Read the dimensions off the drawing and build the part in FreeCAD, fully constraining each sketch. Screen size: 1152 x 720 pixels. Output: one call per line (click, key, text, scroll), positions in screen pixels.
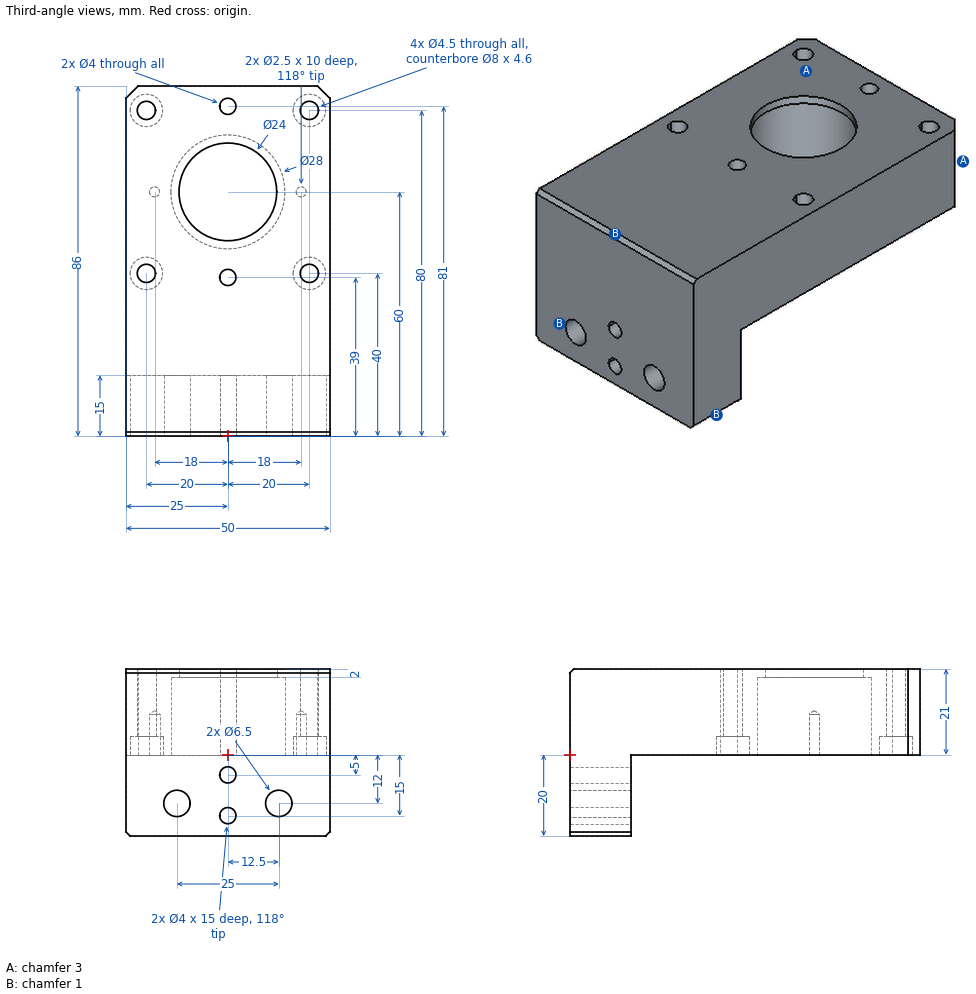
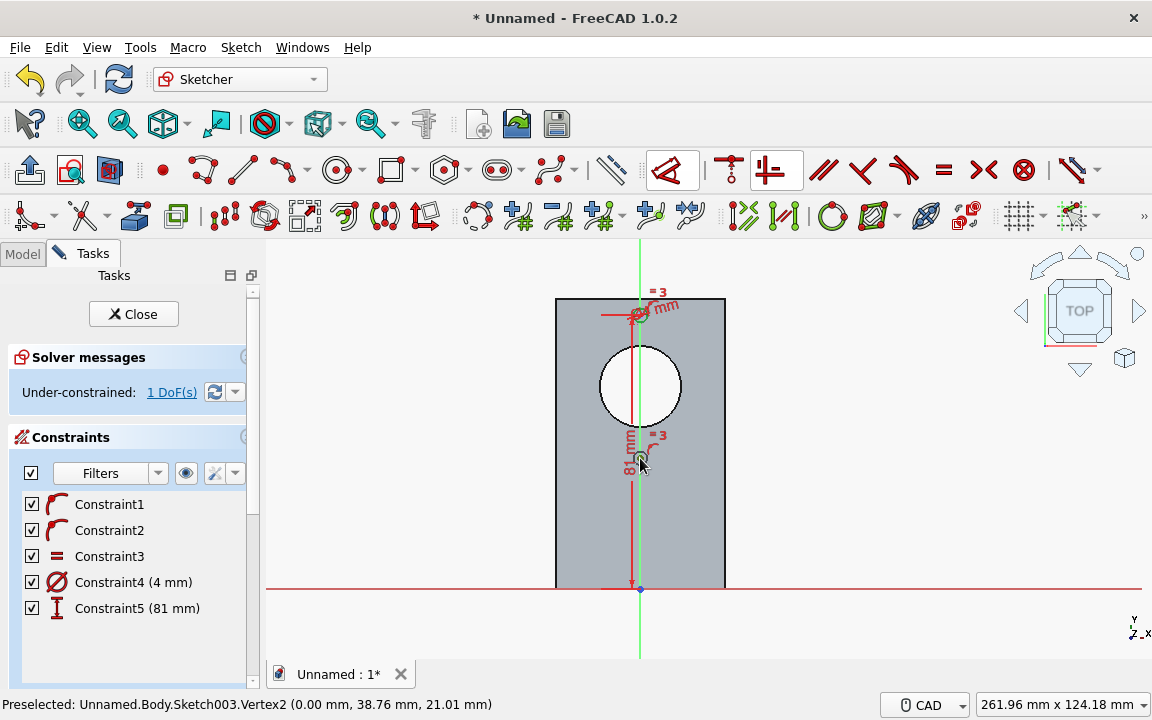
key(i)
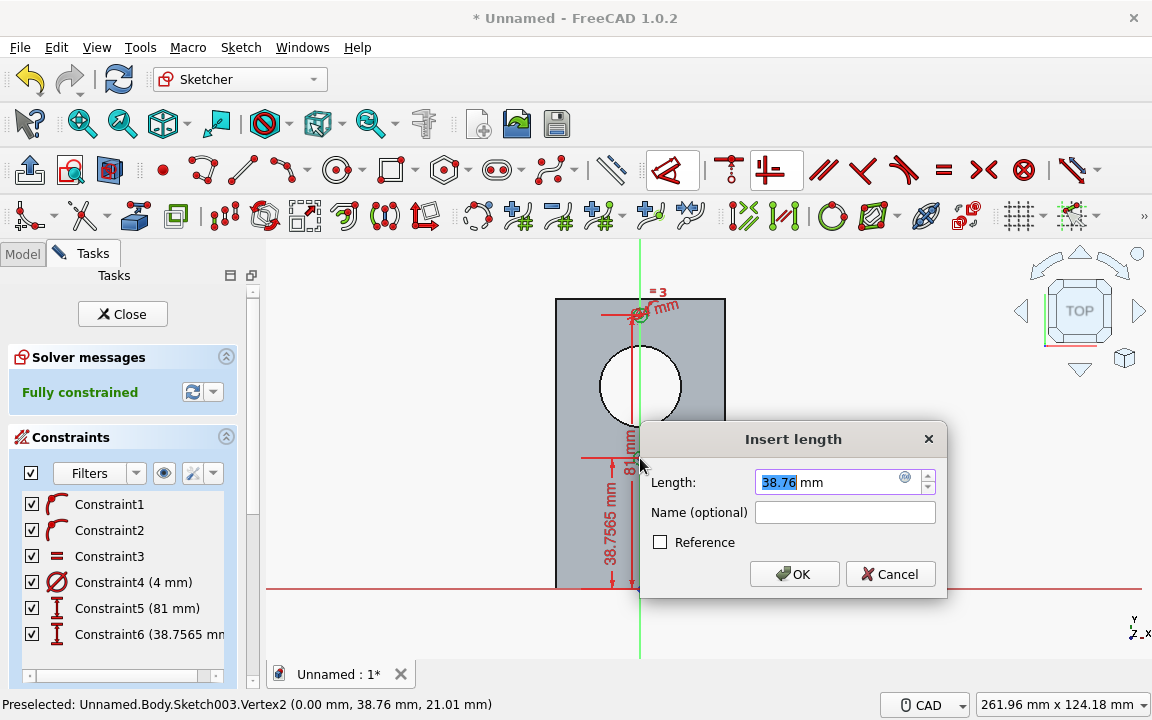
text(39)
key(Return)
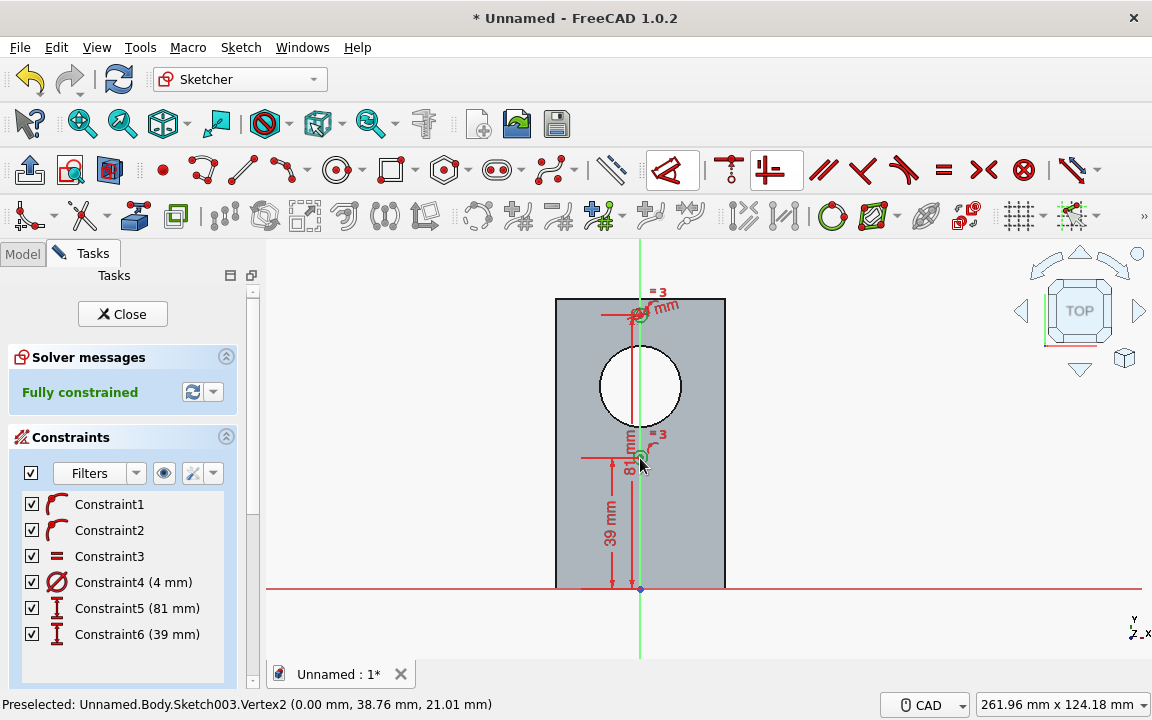
click(123, 314)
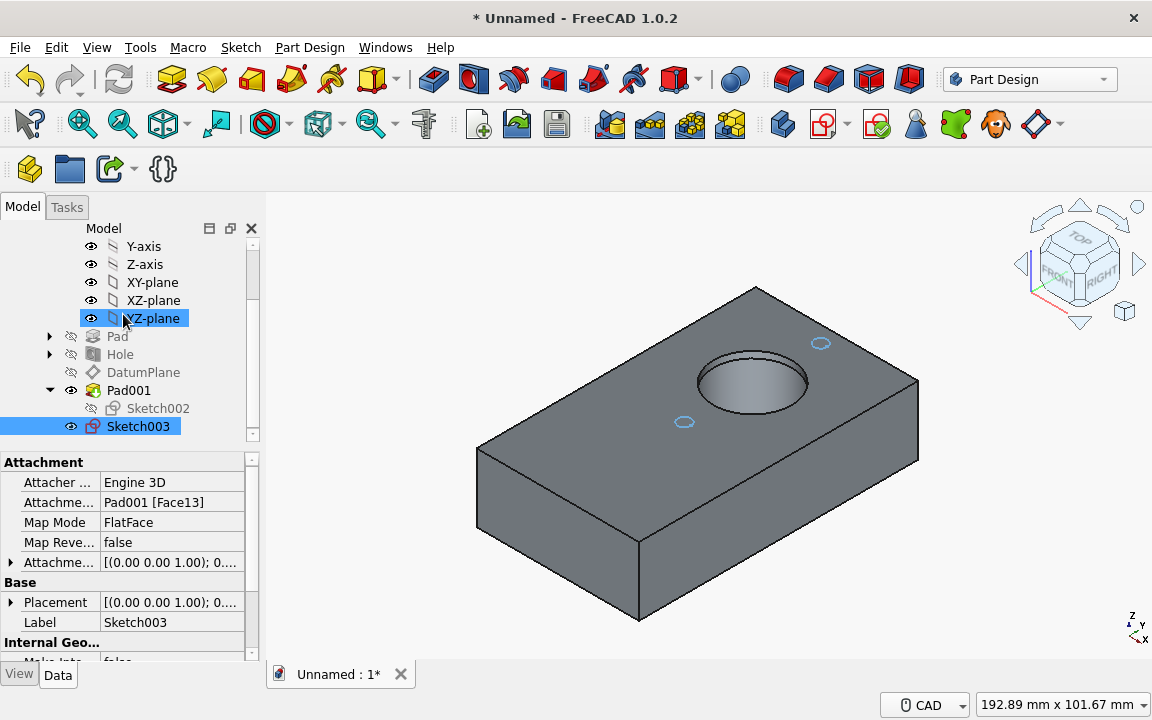
click(474, 80)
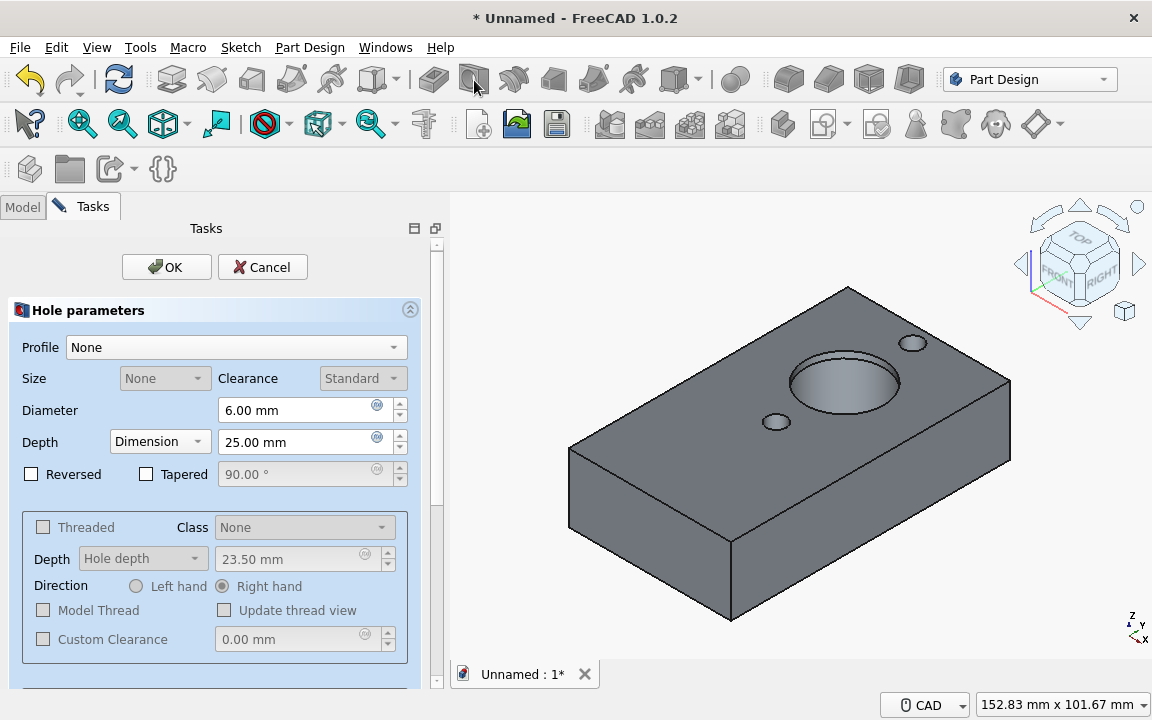
triple_click(305, 410)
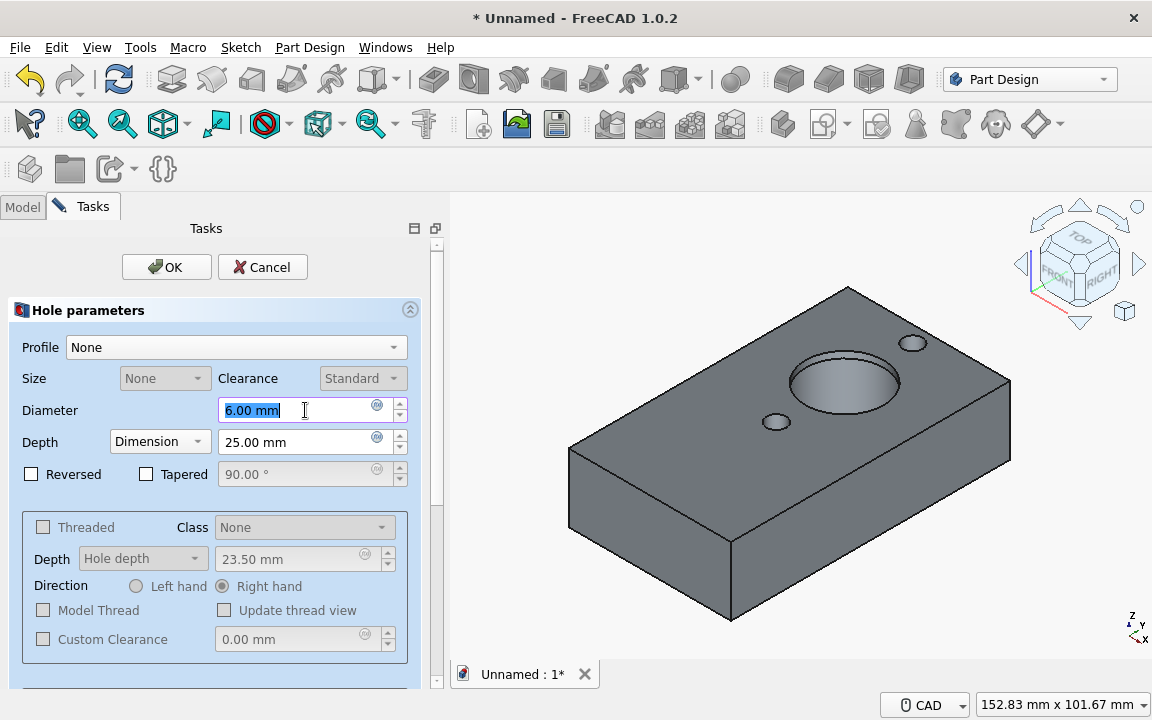
text(4)
key(Tab)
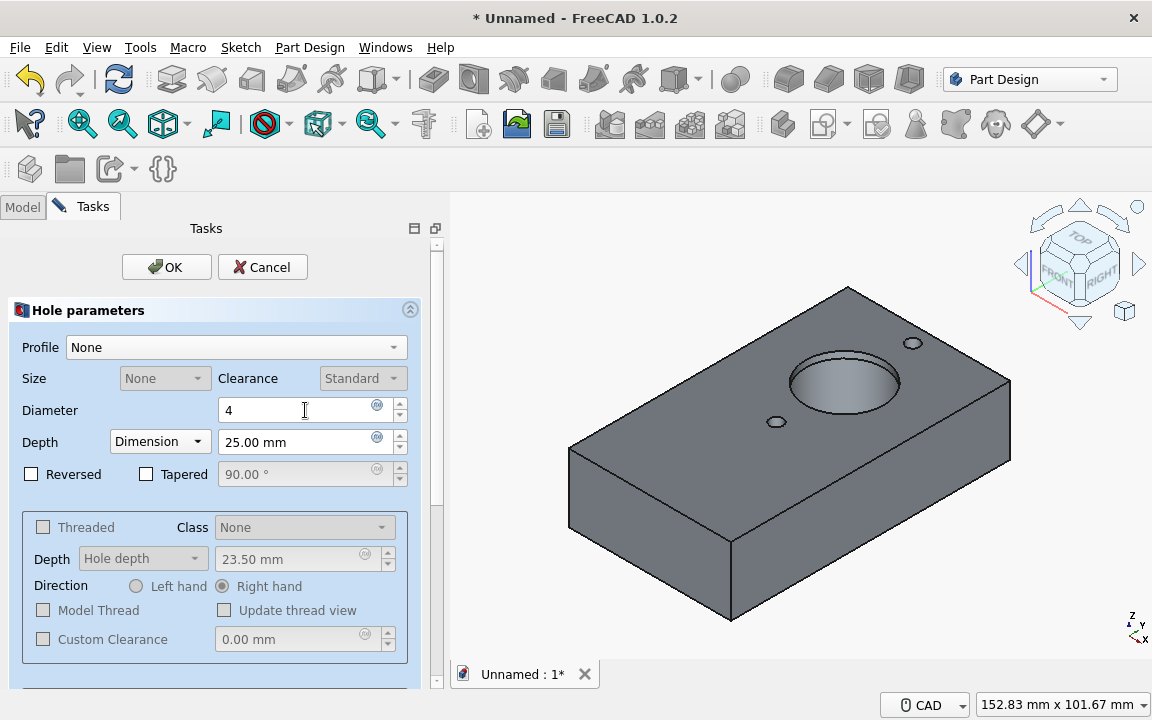
click(161, 442)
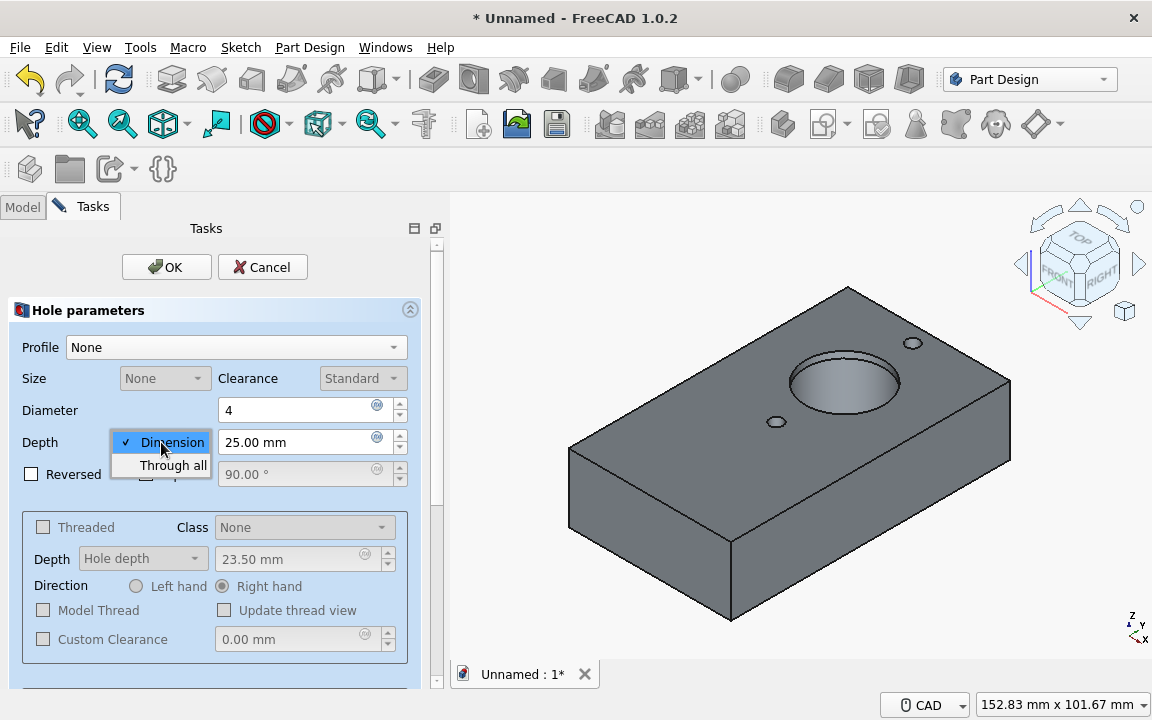
click(160, 466)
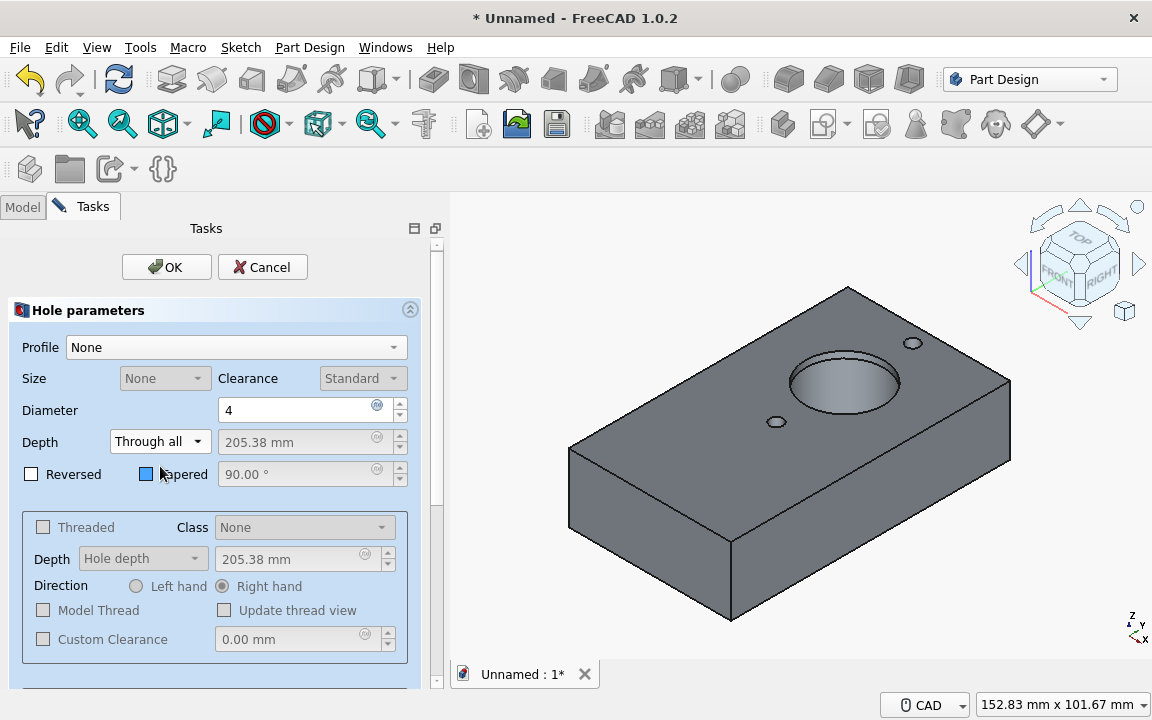
click(167, 267)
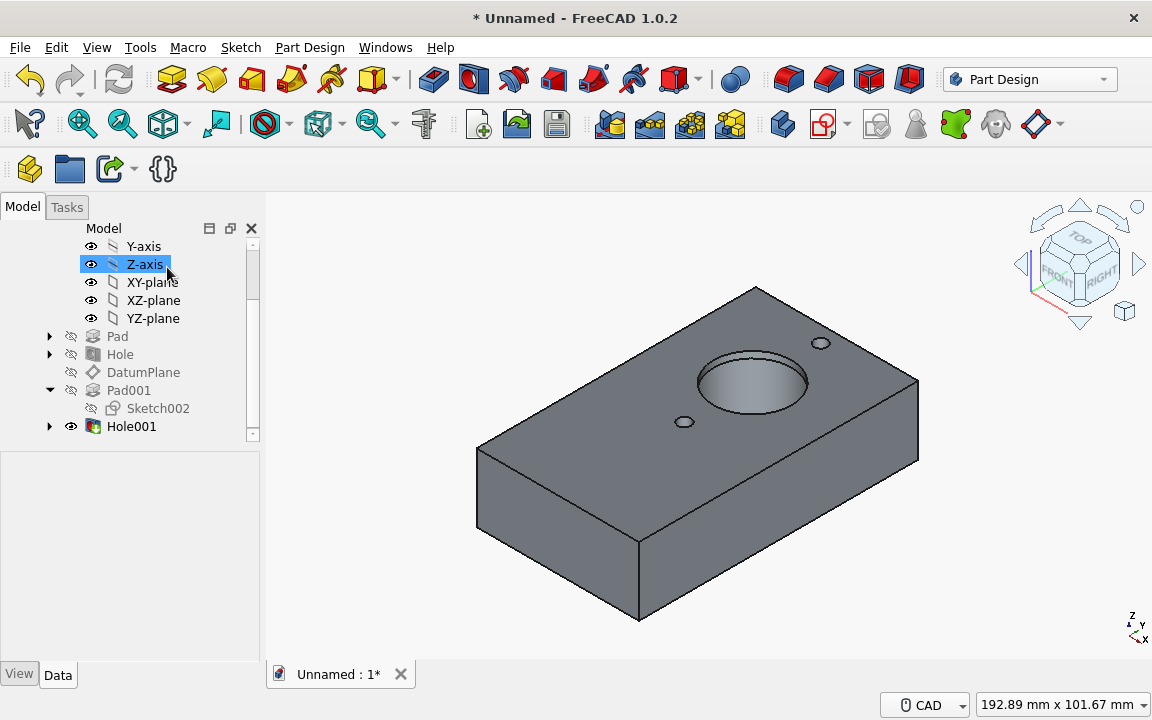
key(5)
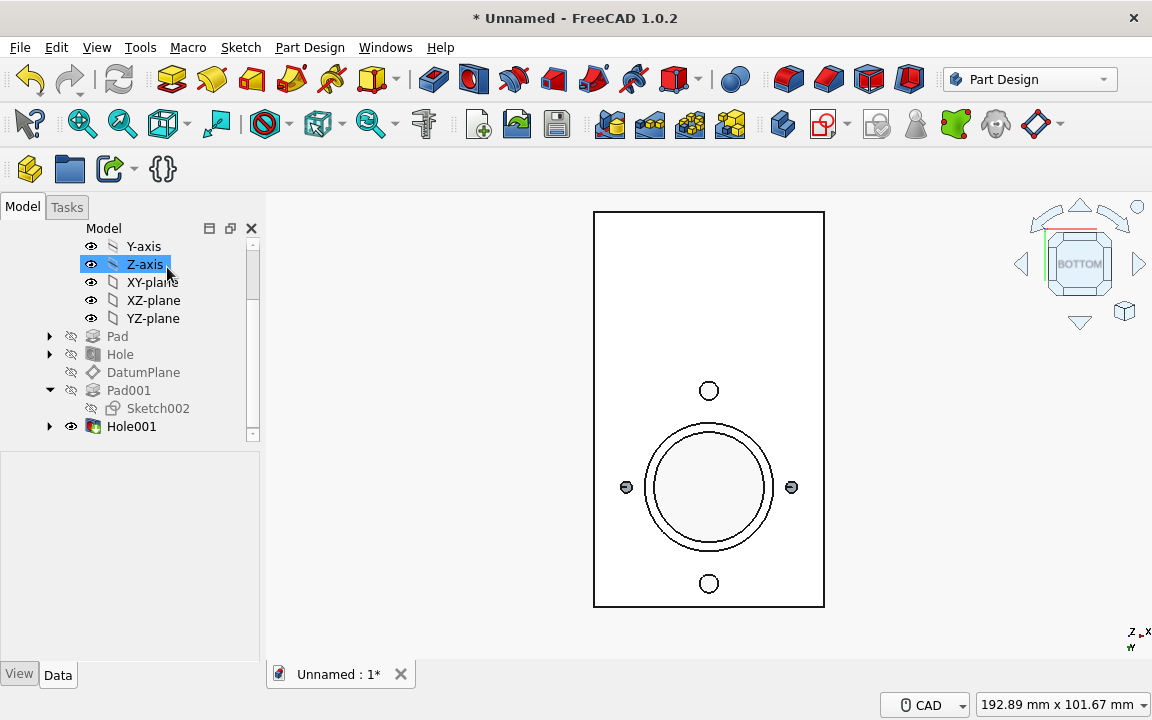
click(709, 295)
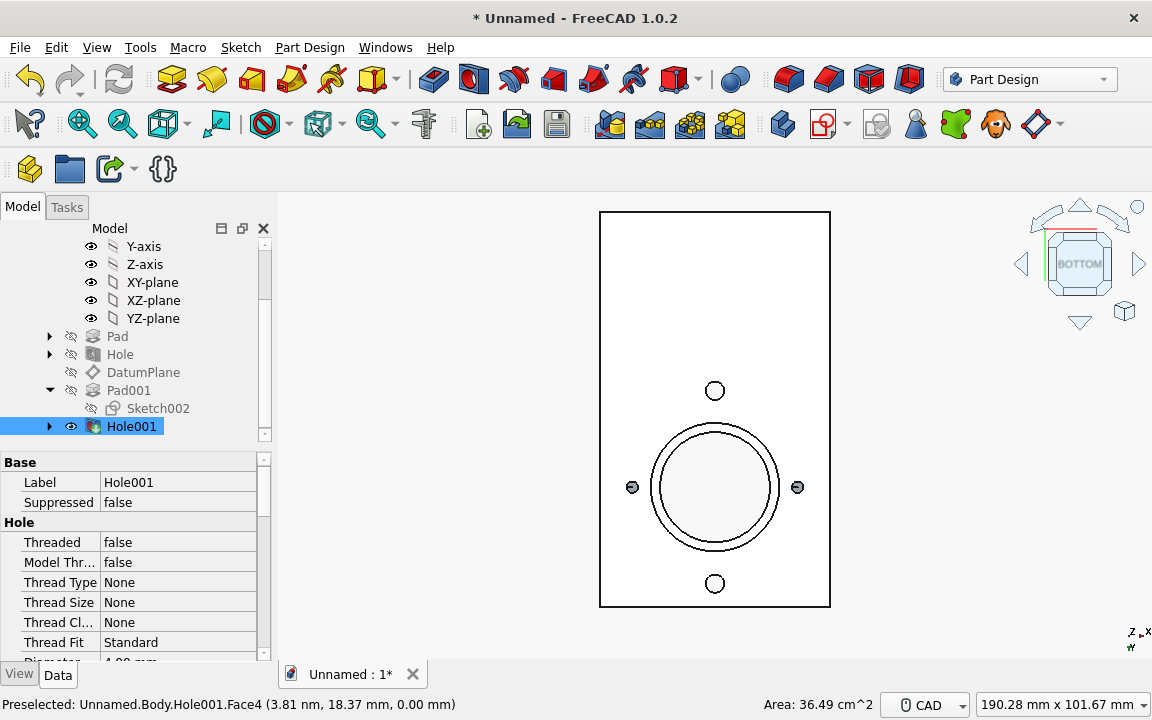
click(824, 124)